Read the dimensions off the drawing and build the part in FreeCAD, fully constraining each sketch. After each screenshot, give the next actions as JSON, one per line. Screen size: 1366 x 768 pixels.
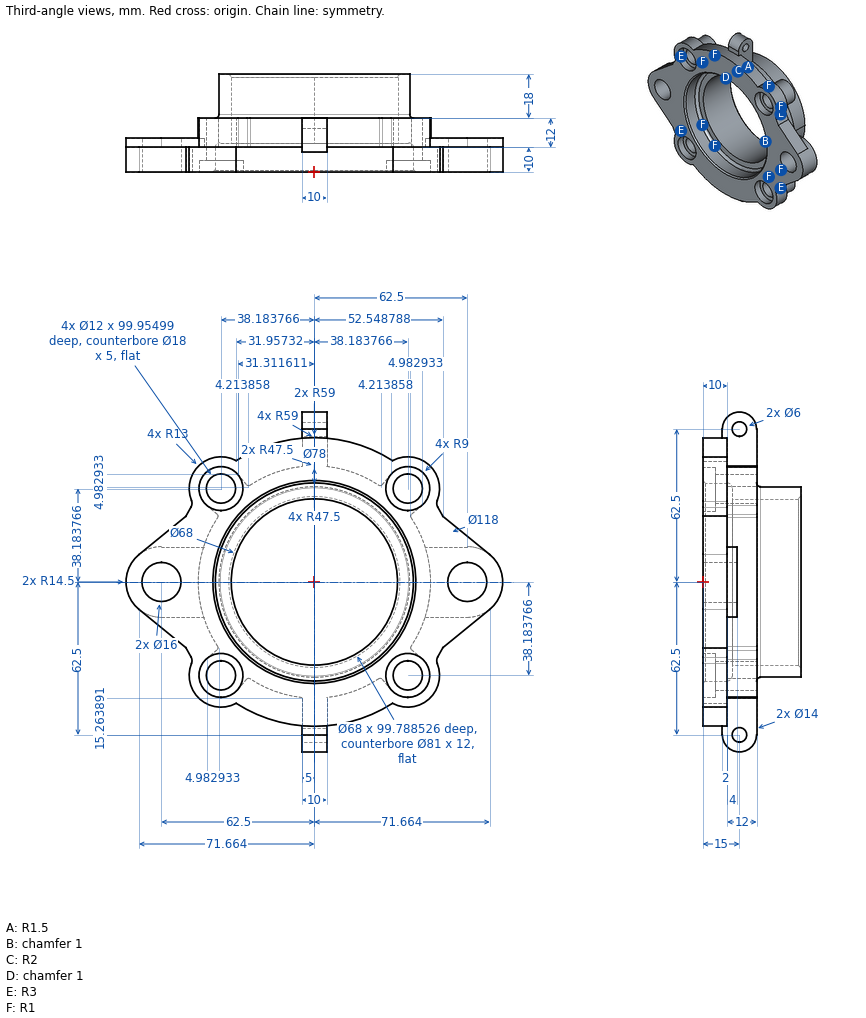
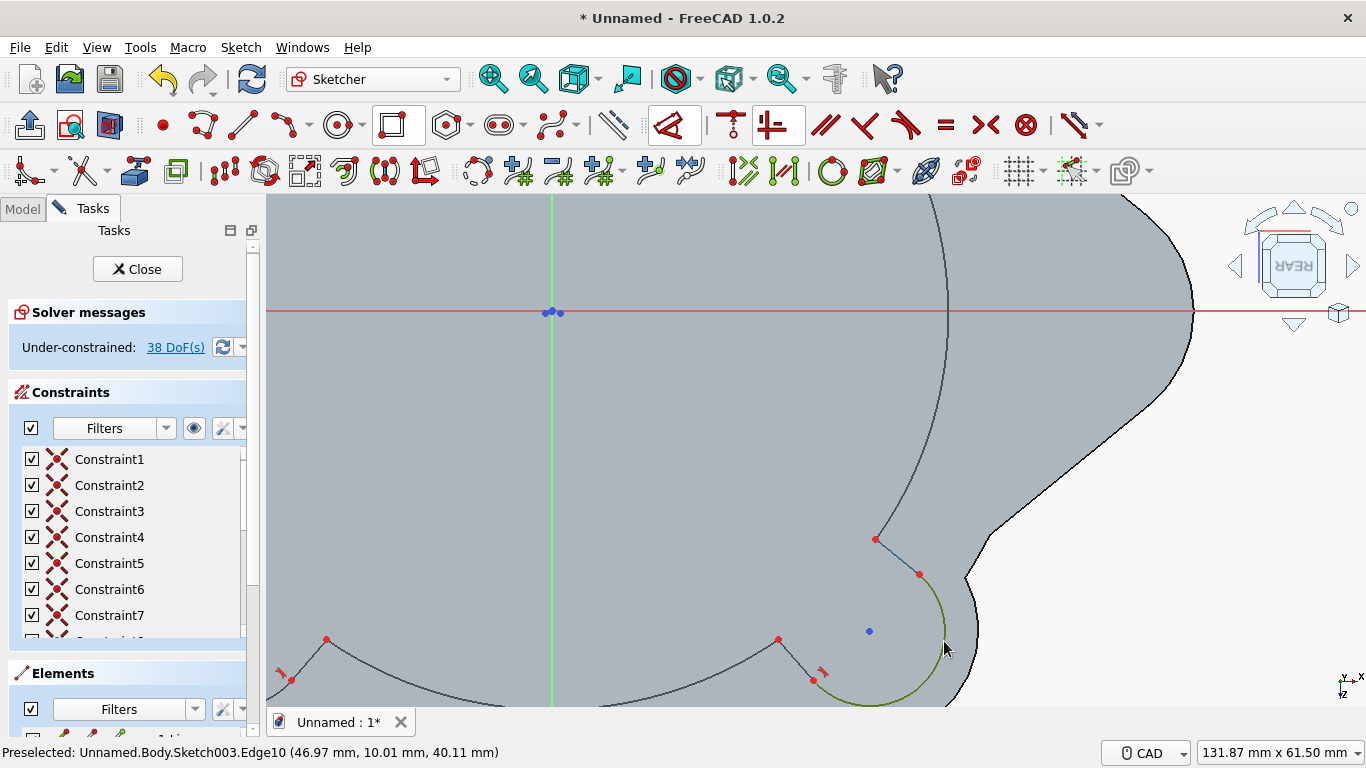
{"action": "left_click", "coordinate": [906, 126]}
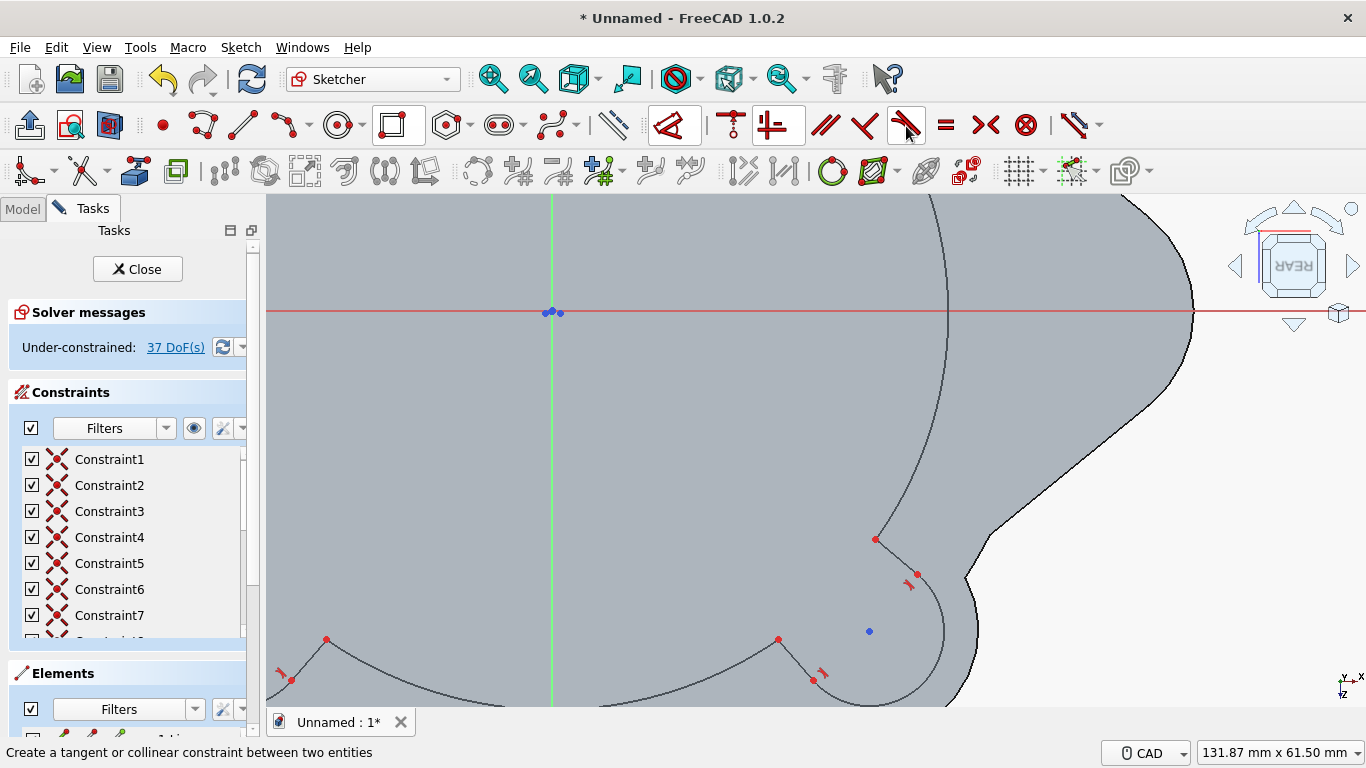
{"action": "scroll", "coordinate": [907, 564], "scroll_direction": "down", "scroll_amount": 4}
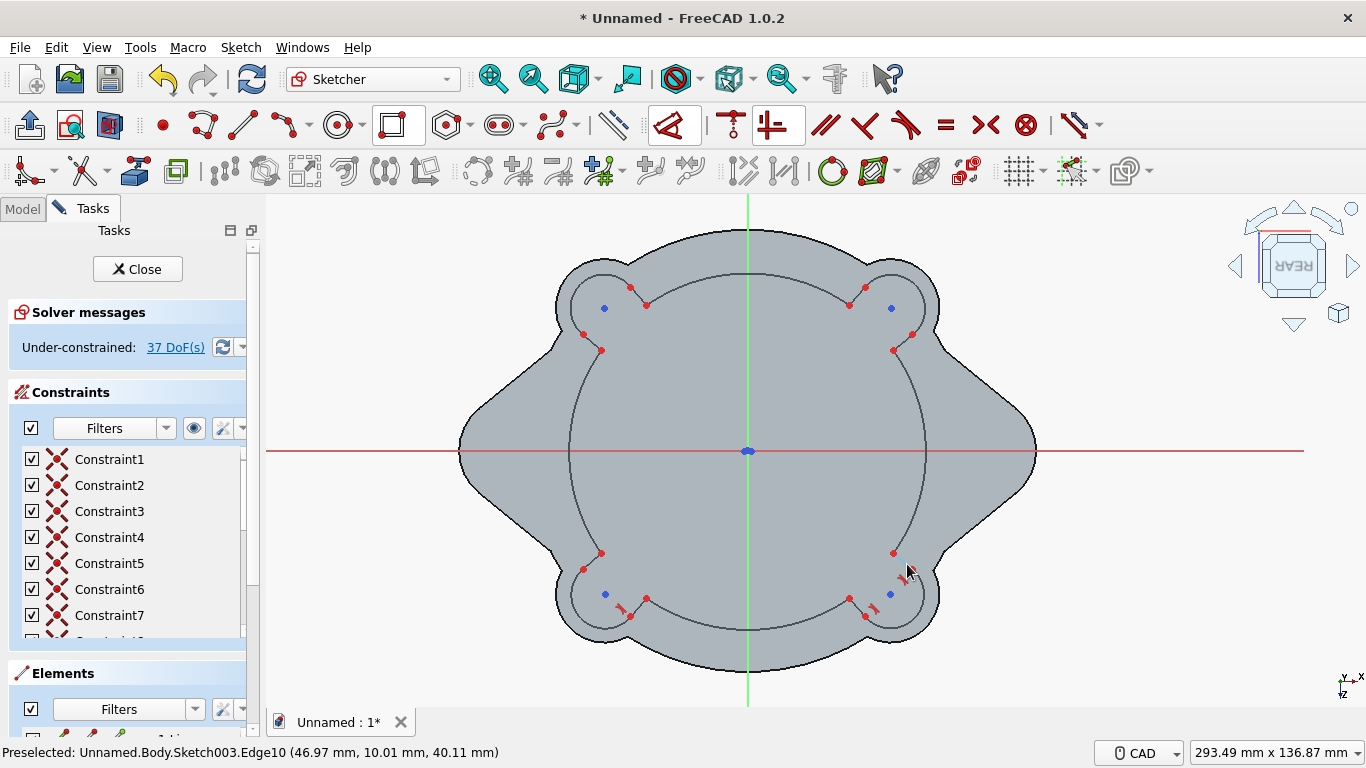
{"action": "scroll", "coordinate": [899, 346], "scroll_direction": "up", "scroll_amount": 4}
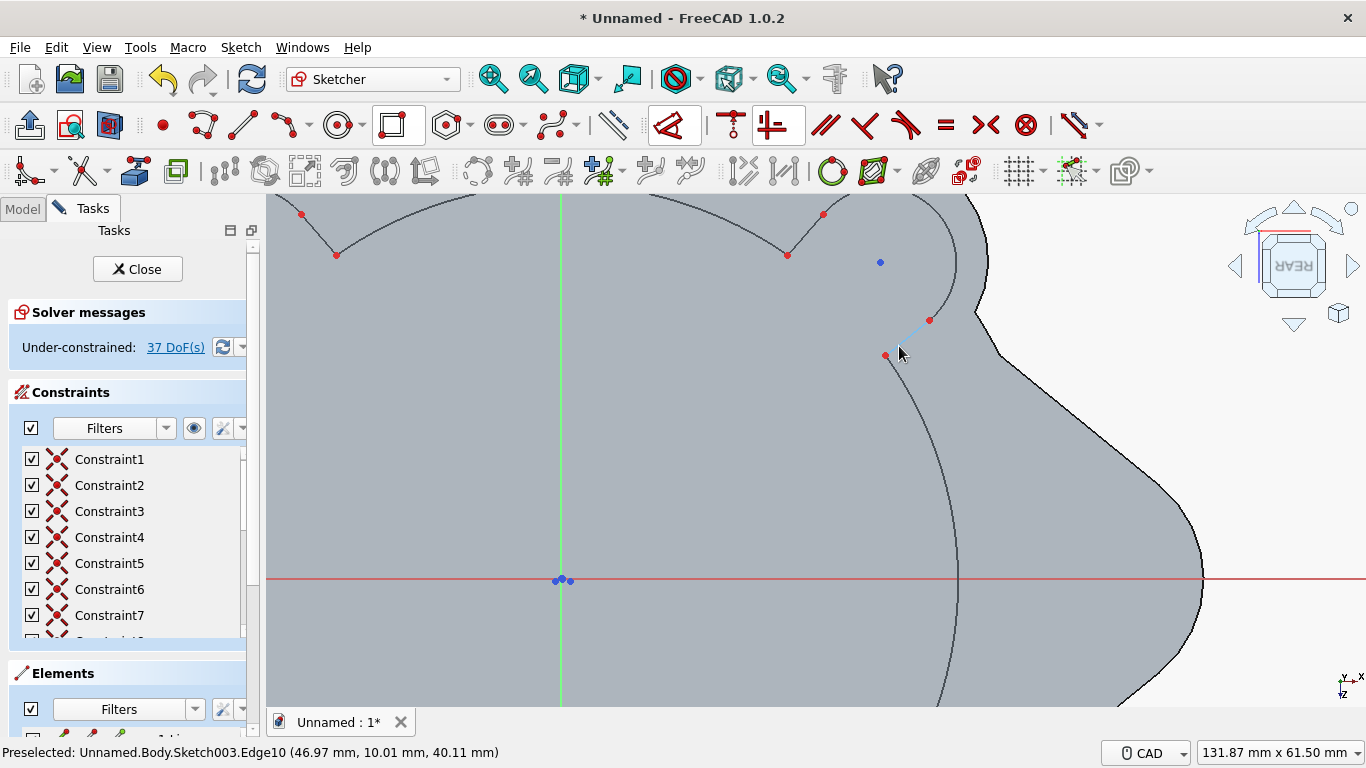
{"action": "left_click", "coordinate": [899, 345]}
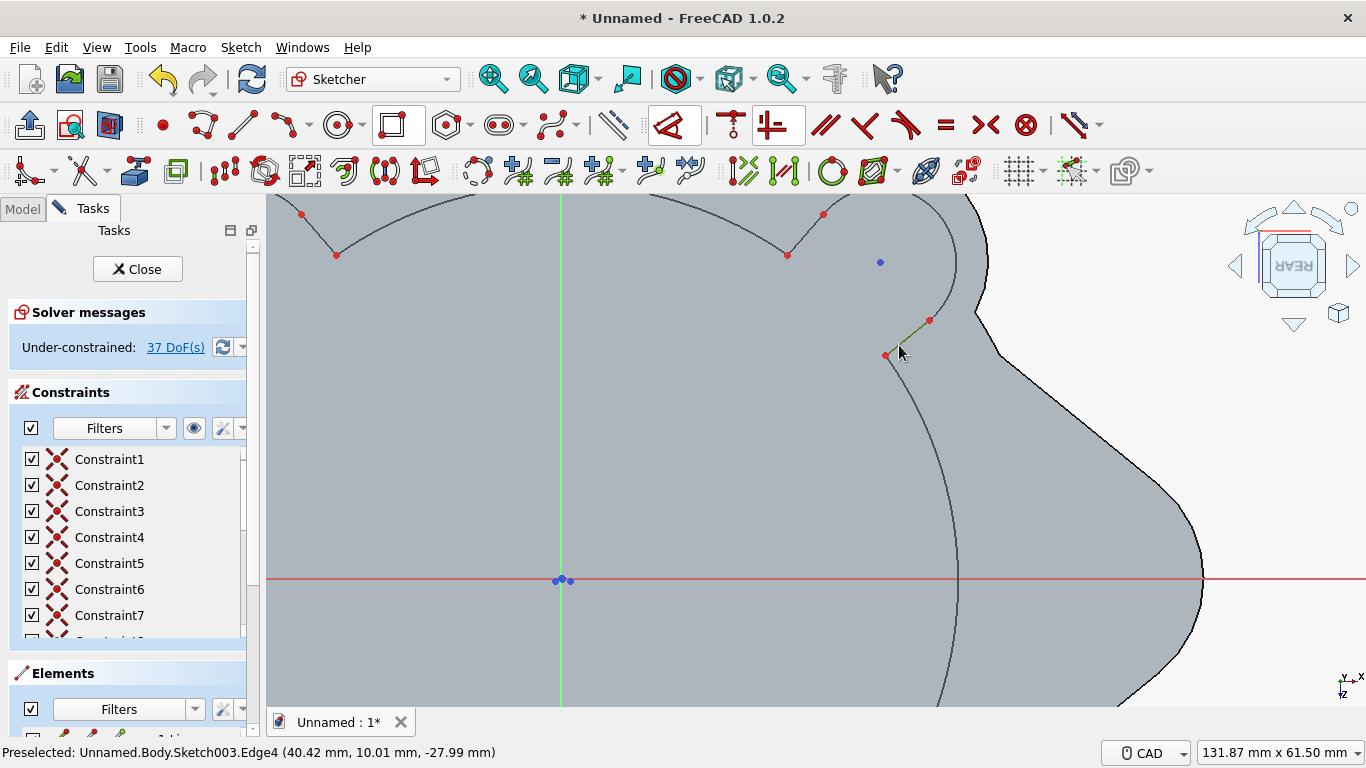
{"action": "left_click", "coordinate": [956, 254]}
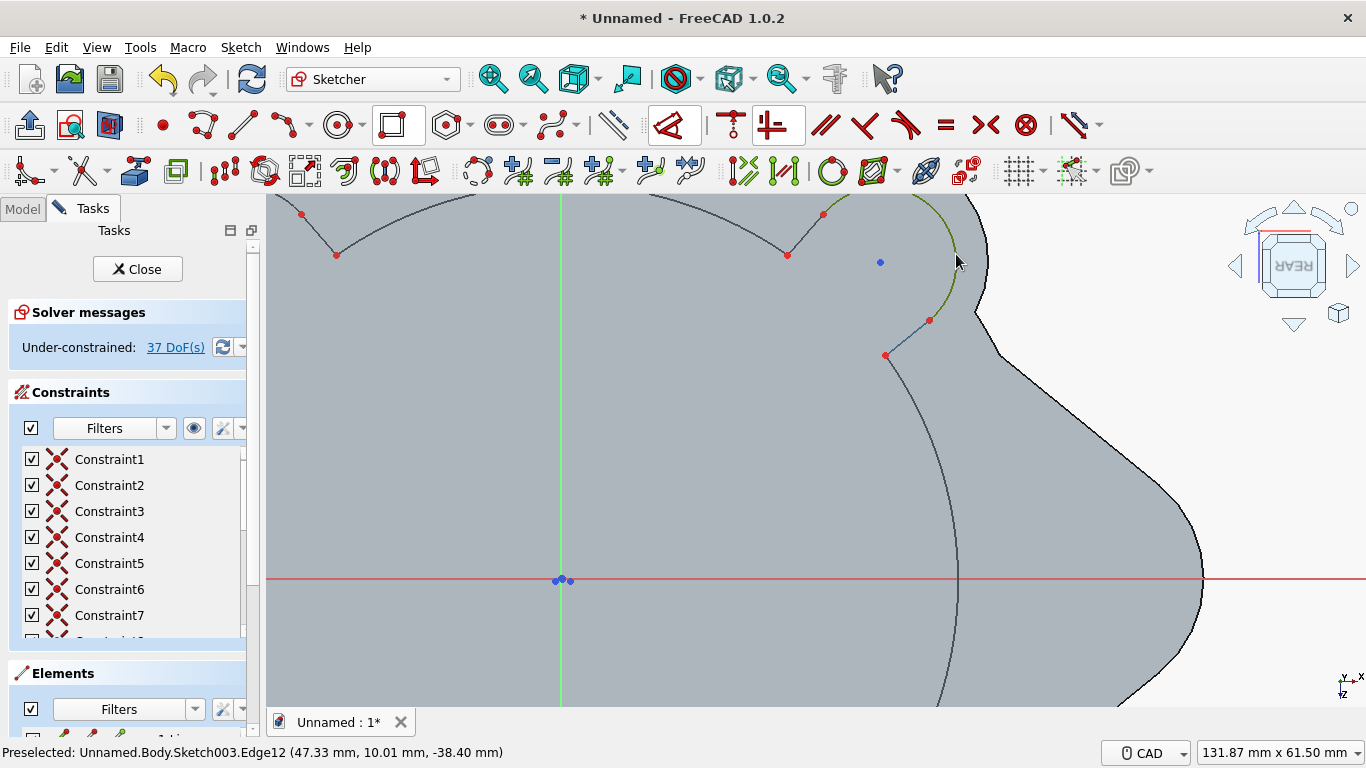
{"action": "left_click", "coordinate": [906, 126]}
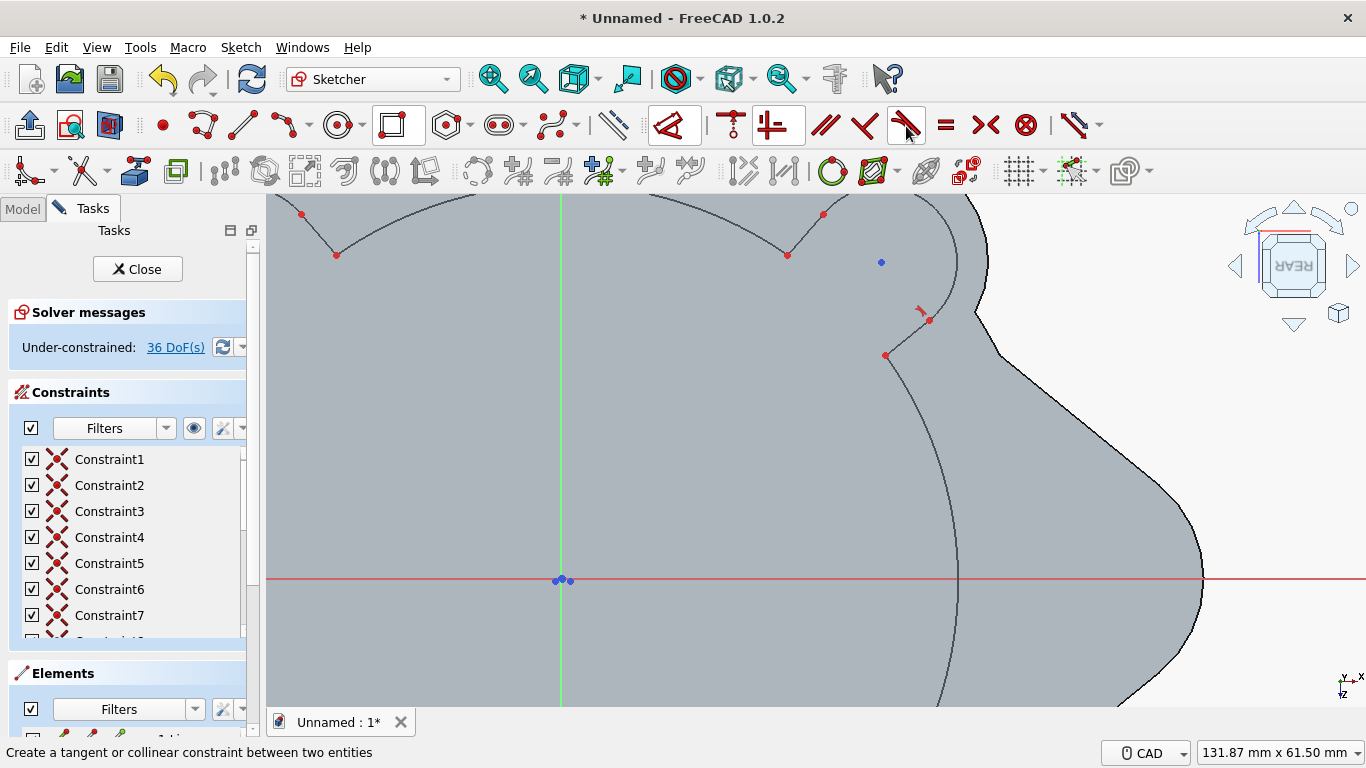
{"action": "left_click", "coordinate": [813, 227]}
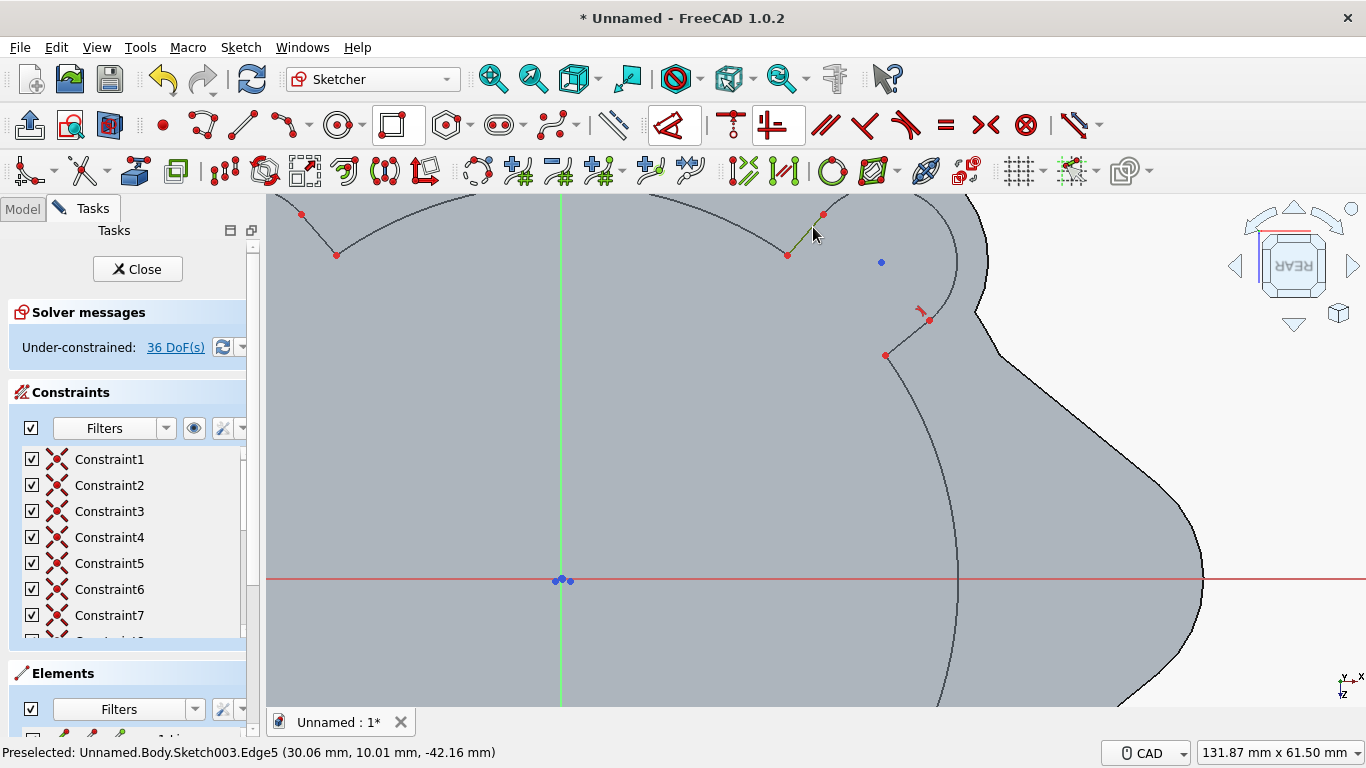
{"action": "left_click", "coordinate": [957, 253]}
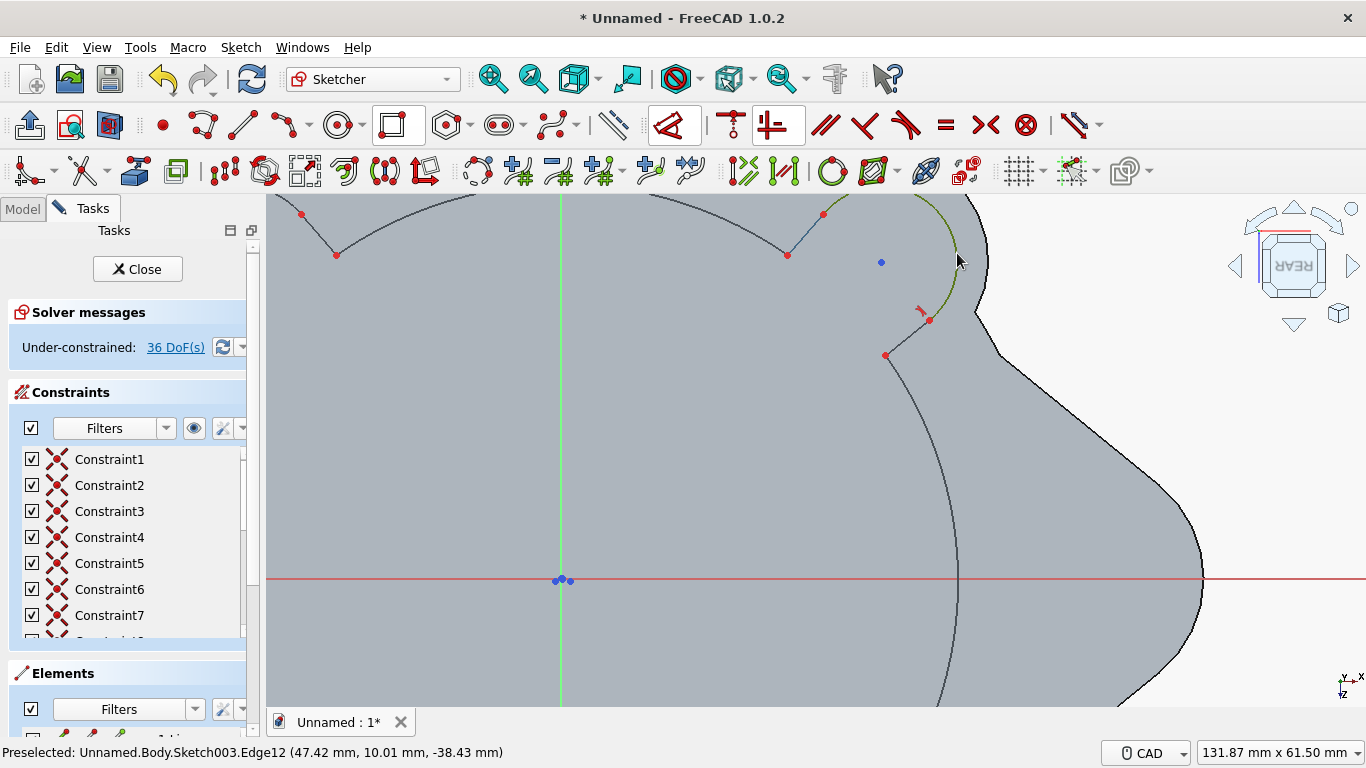
{"action": "left_click", "coordinate": [906, 126]}